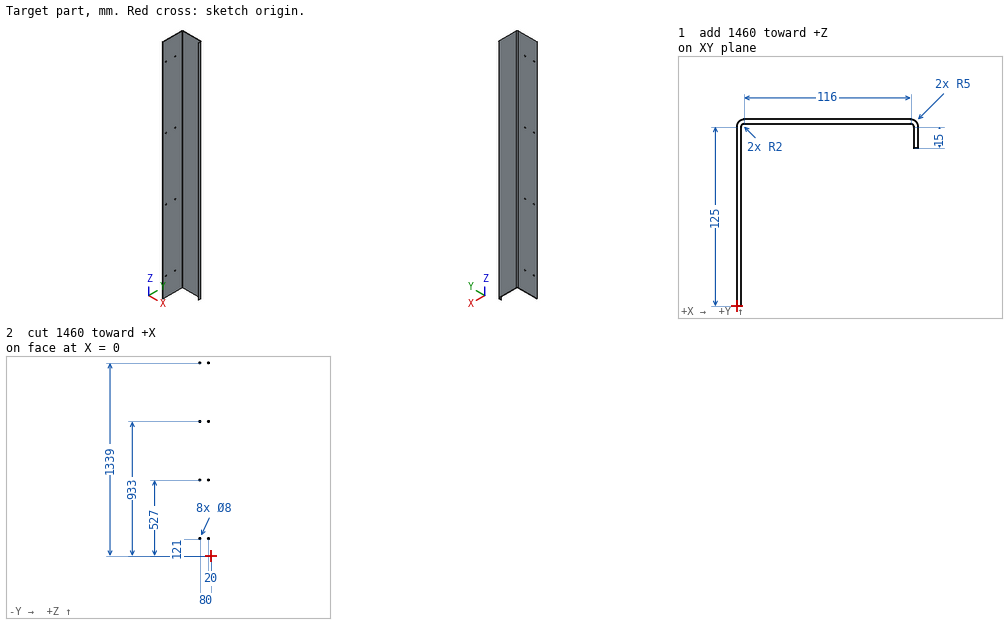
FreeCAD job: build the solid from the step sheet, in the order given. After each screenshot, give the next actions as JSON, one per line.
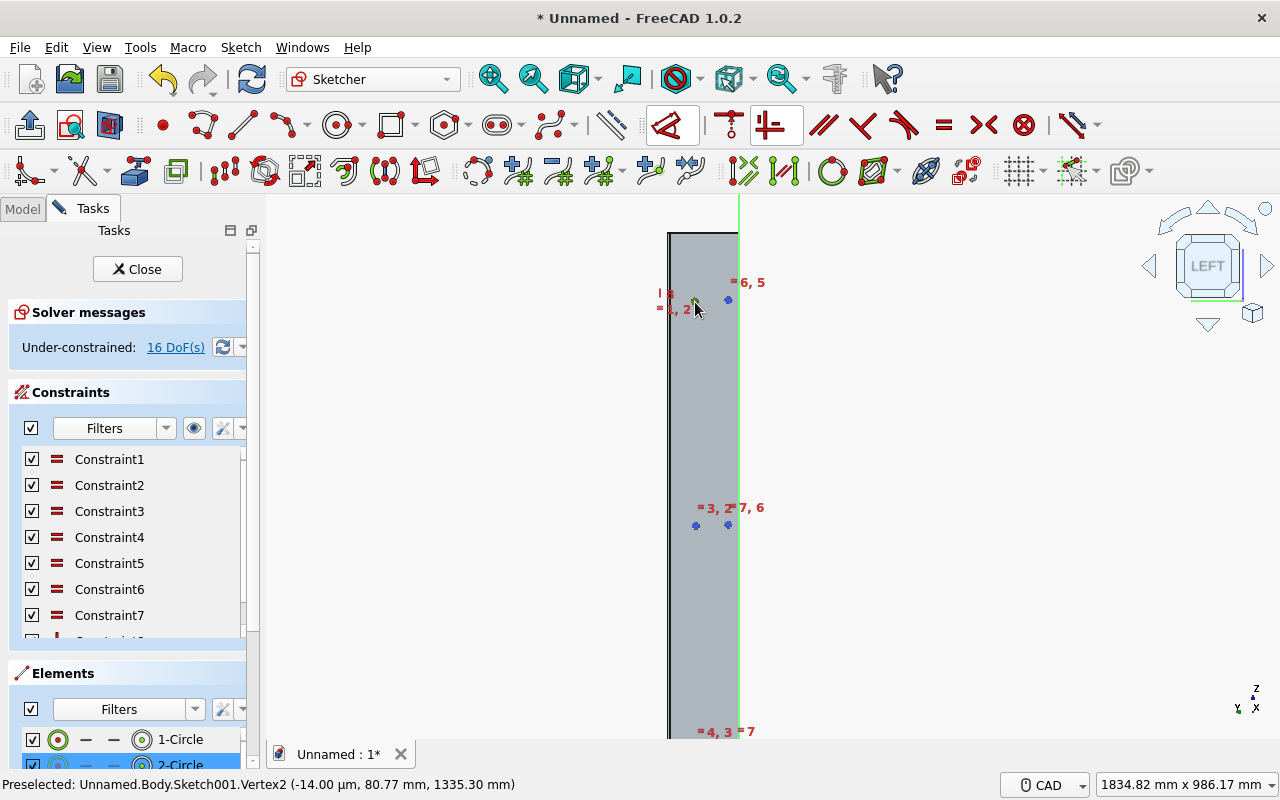
{"action": "left_click", "coordinate": [696, 526]}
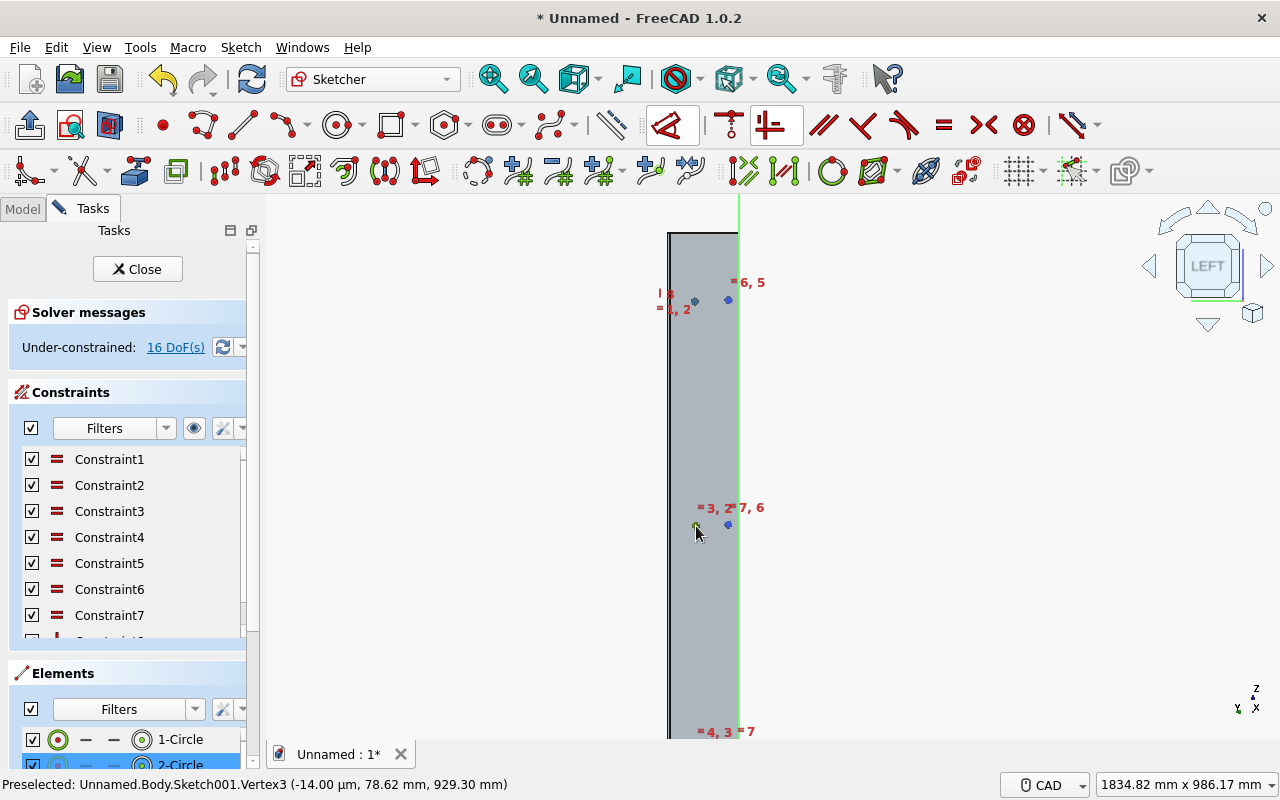
{"action": "key", "text": "v"}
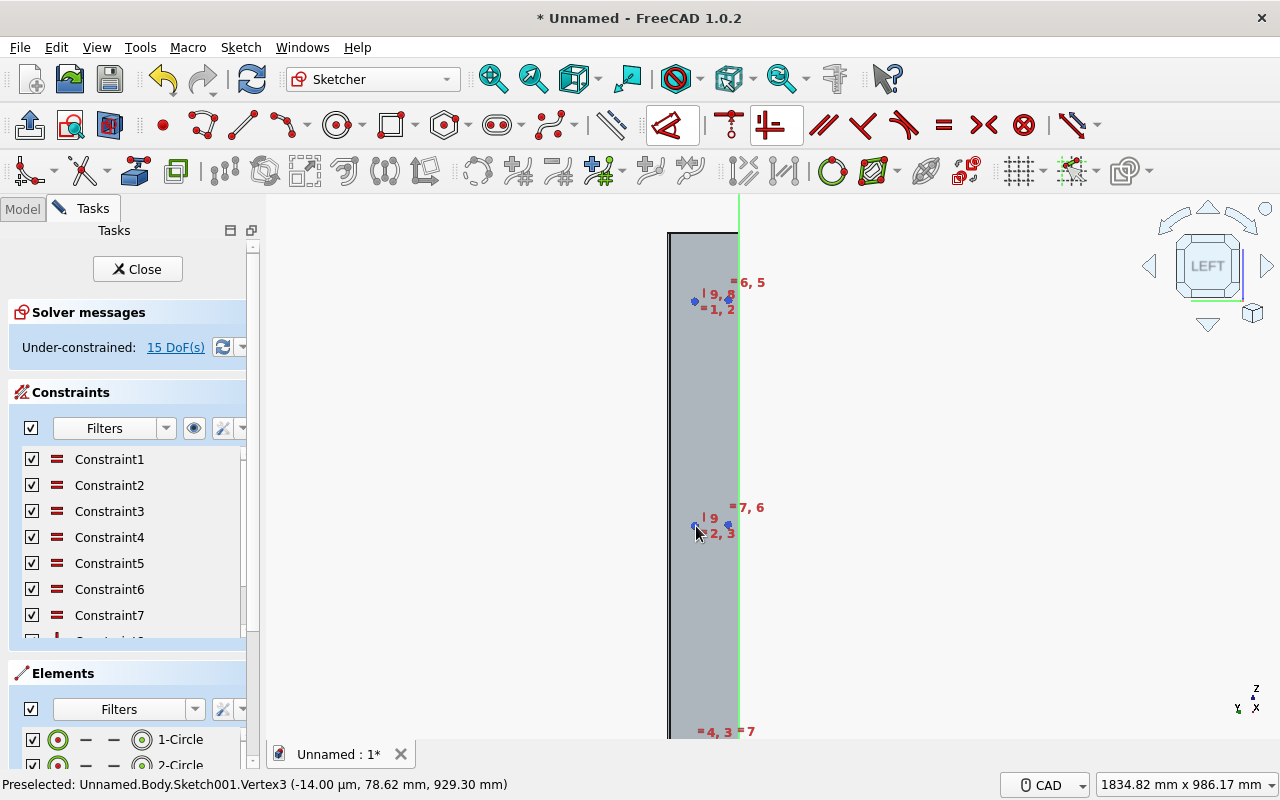
{"action": "scroll", "coordinate": [695, 302], "scroll_direction": "down", "scroll_amount": 4}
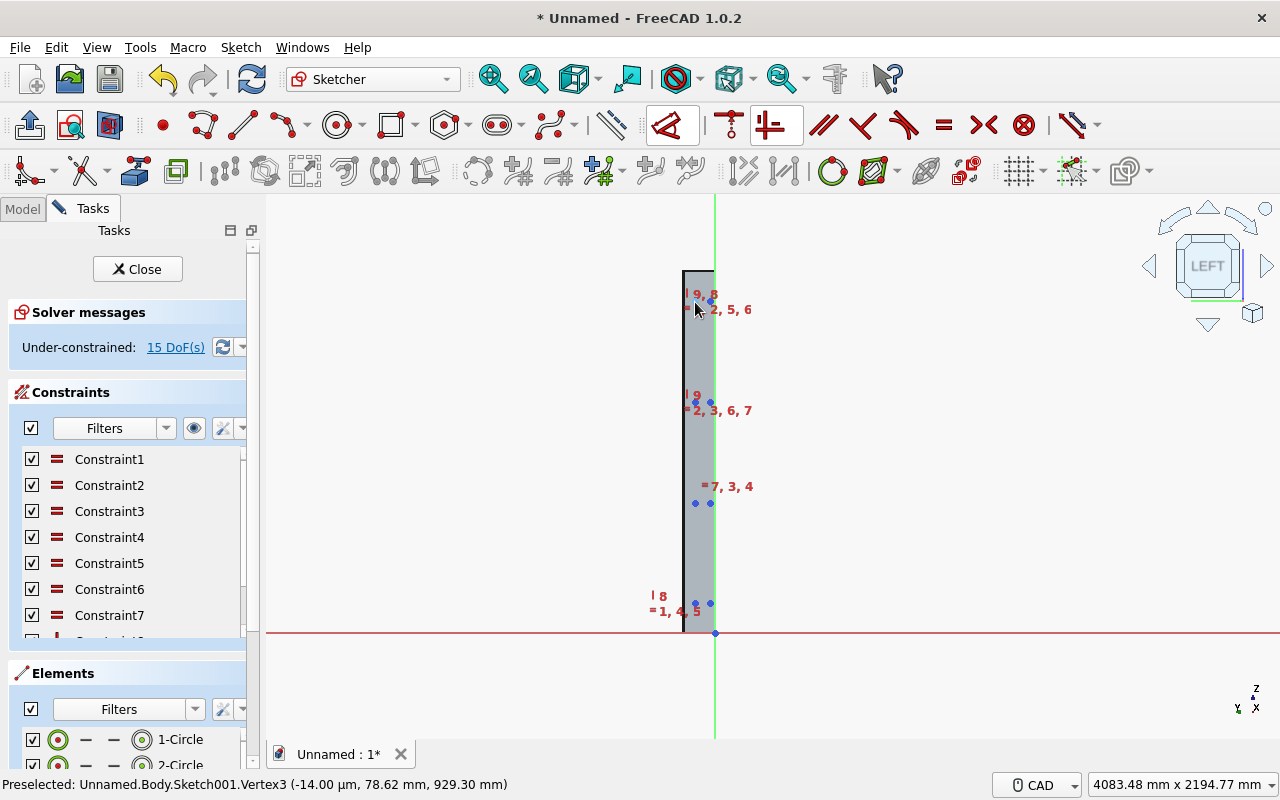
{"action": "left_click", "coordinate": [695, 604]}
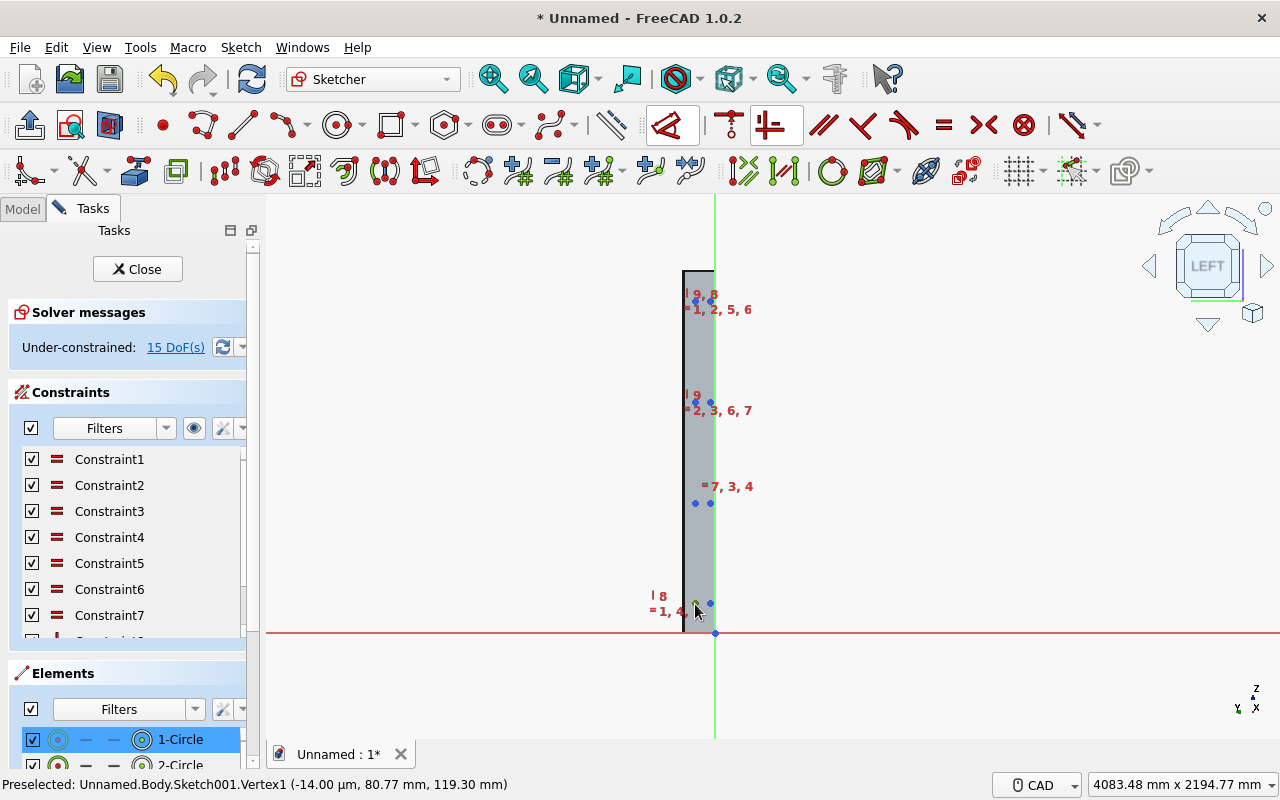
{"action": "left_click", "coordinate": [696, 503]}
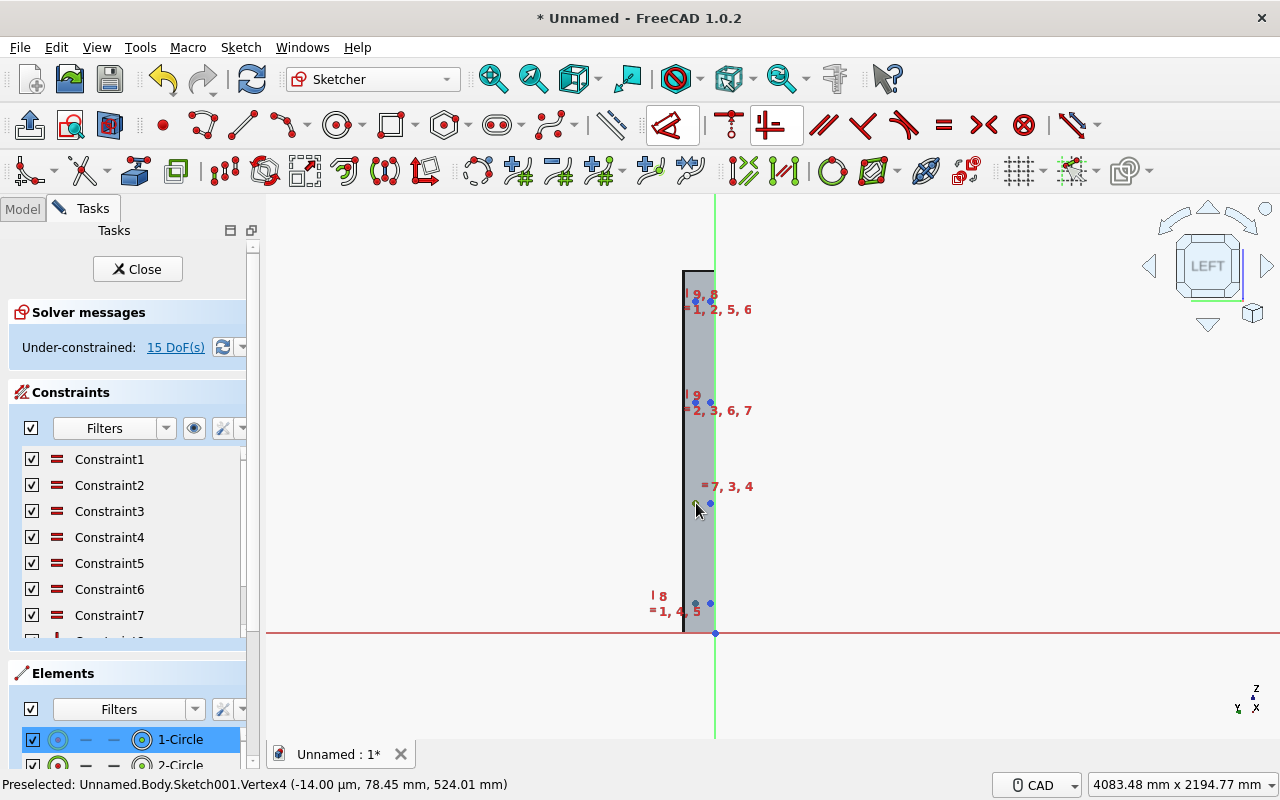
{"action": "key", "text": "v"}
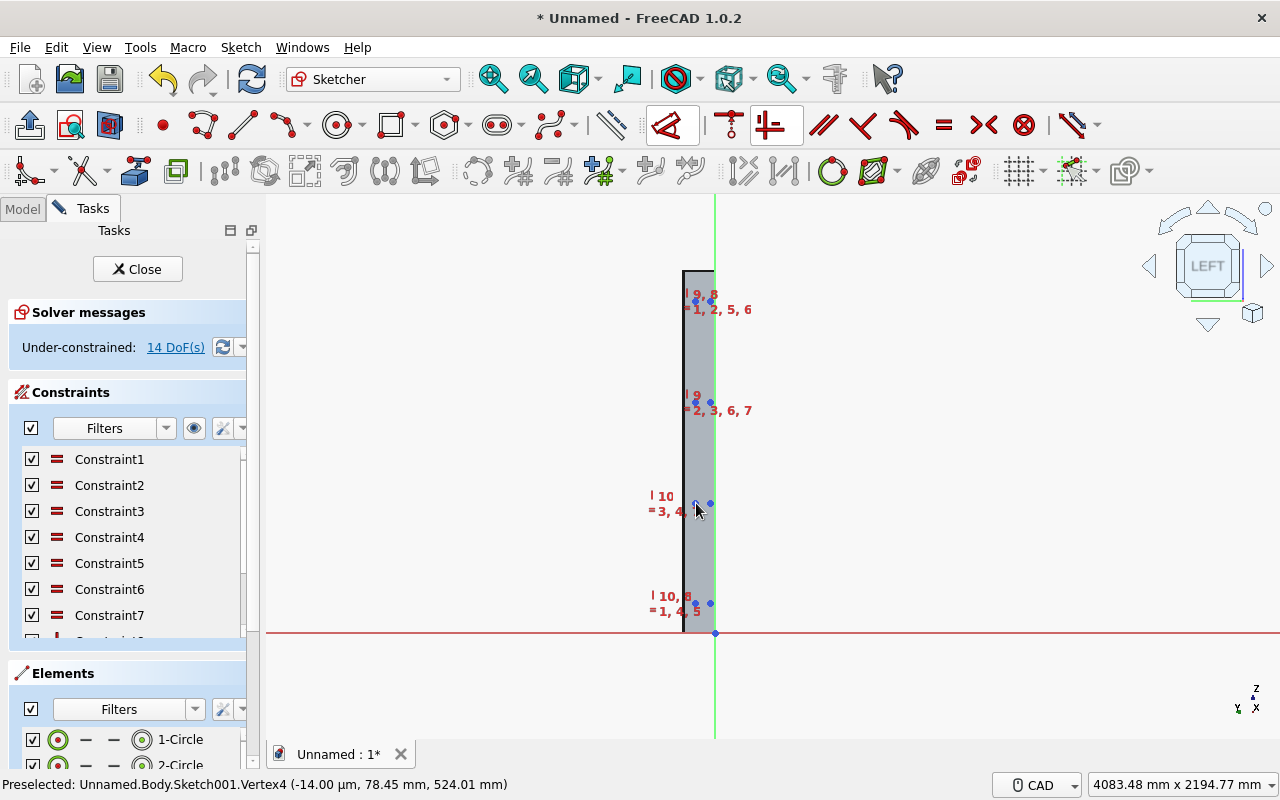
{"action": "left_click", "coordinate": [695, 604]}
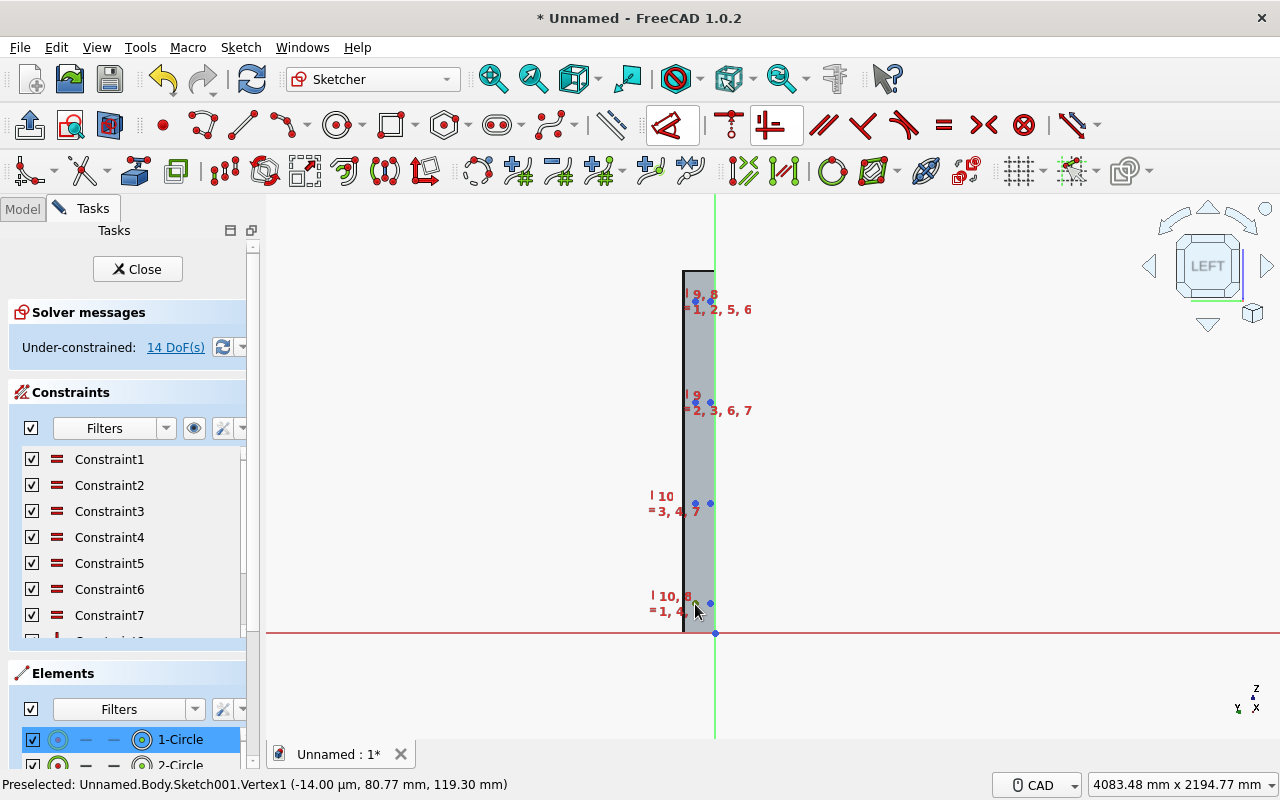
{"action": "left_click", "coordinate": [710, 604]}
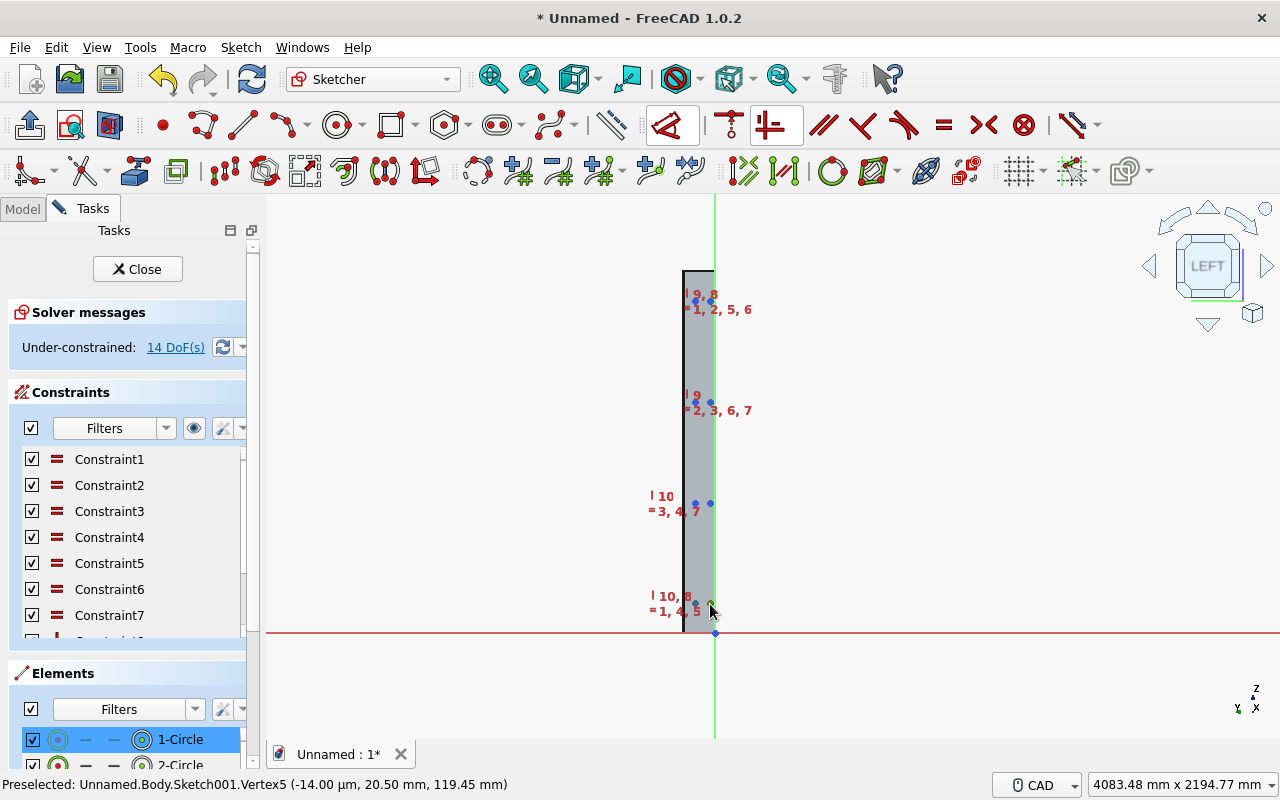
{"action": "left_click", "coordinate": [798, 126]}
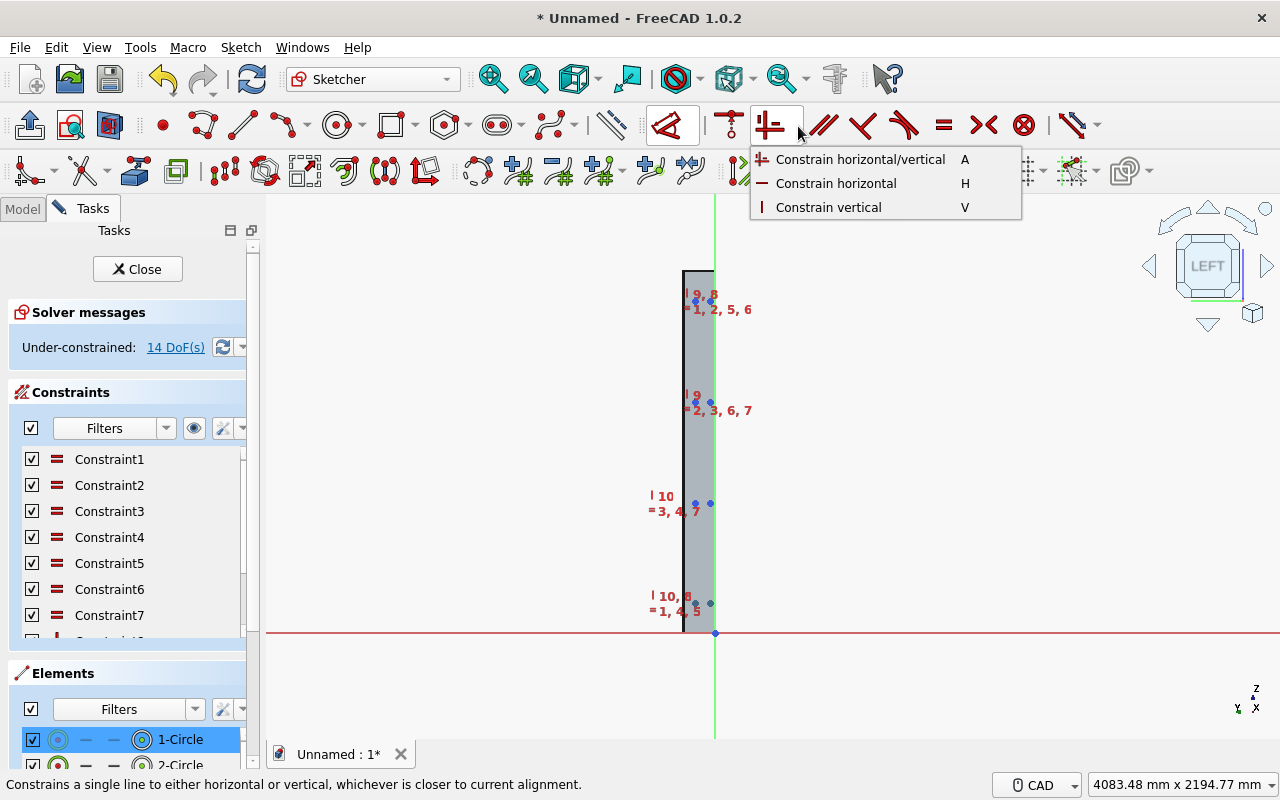
{"action": "left_click", "coordinate": [886, 183]}